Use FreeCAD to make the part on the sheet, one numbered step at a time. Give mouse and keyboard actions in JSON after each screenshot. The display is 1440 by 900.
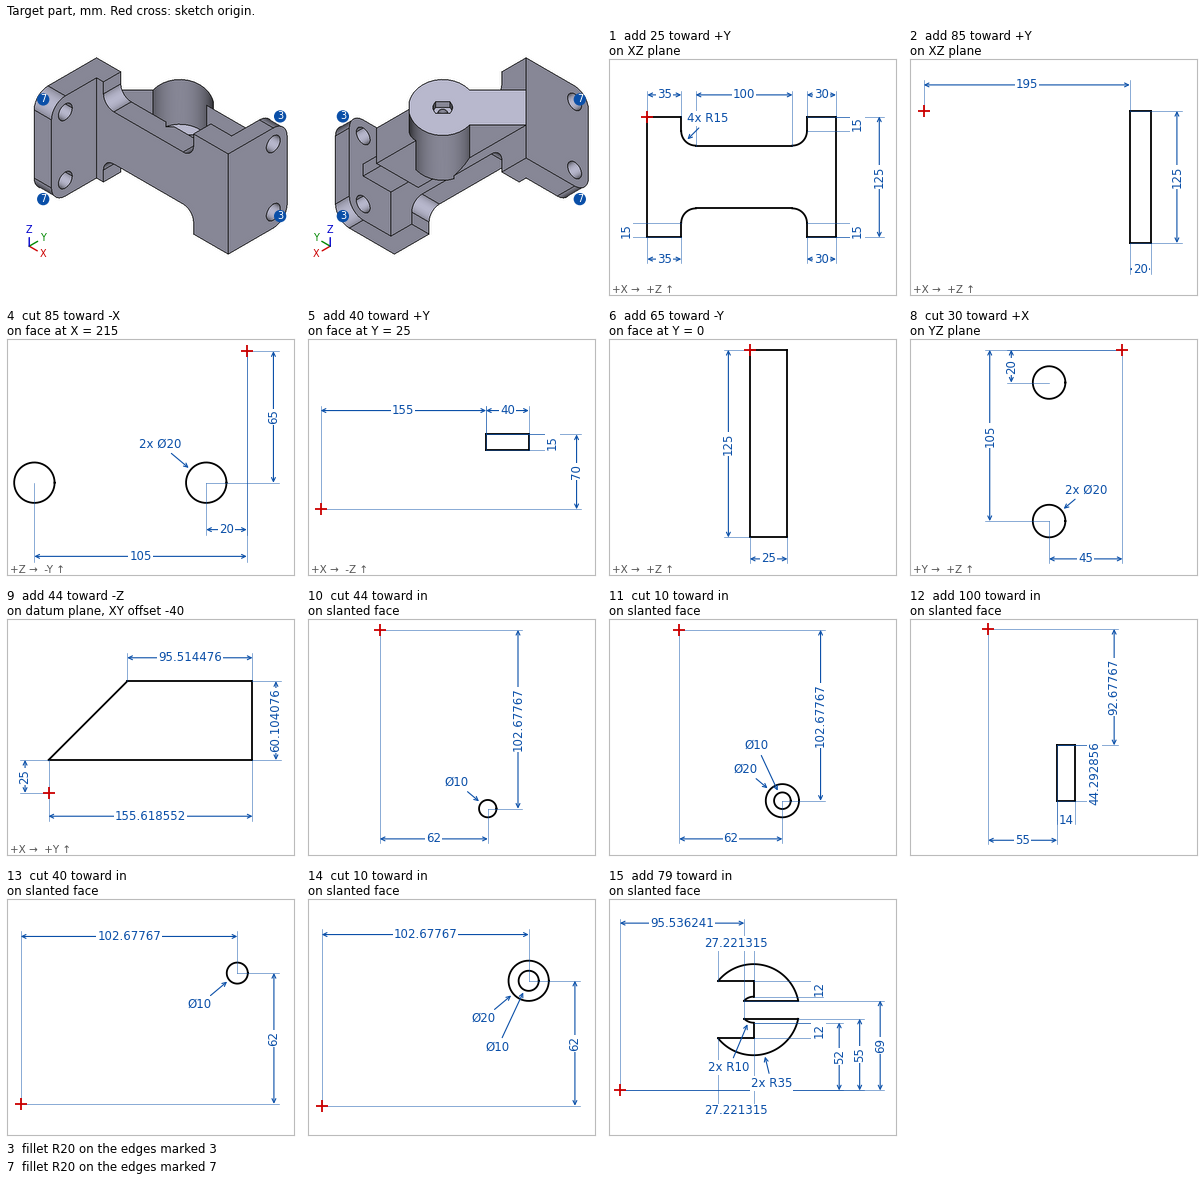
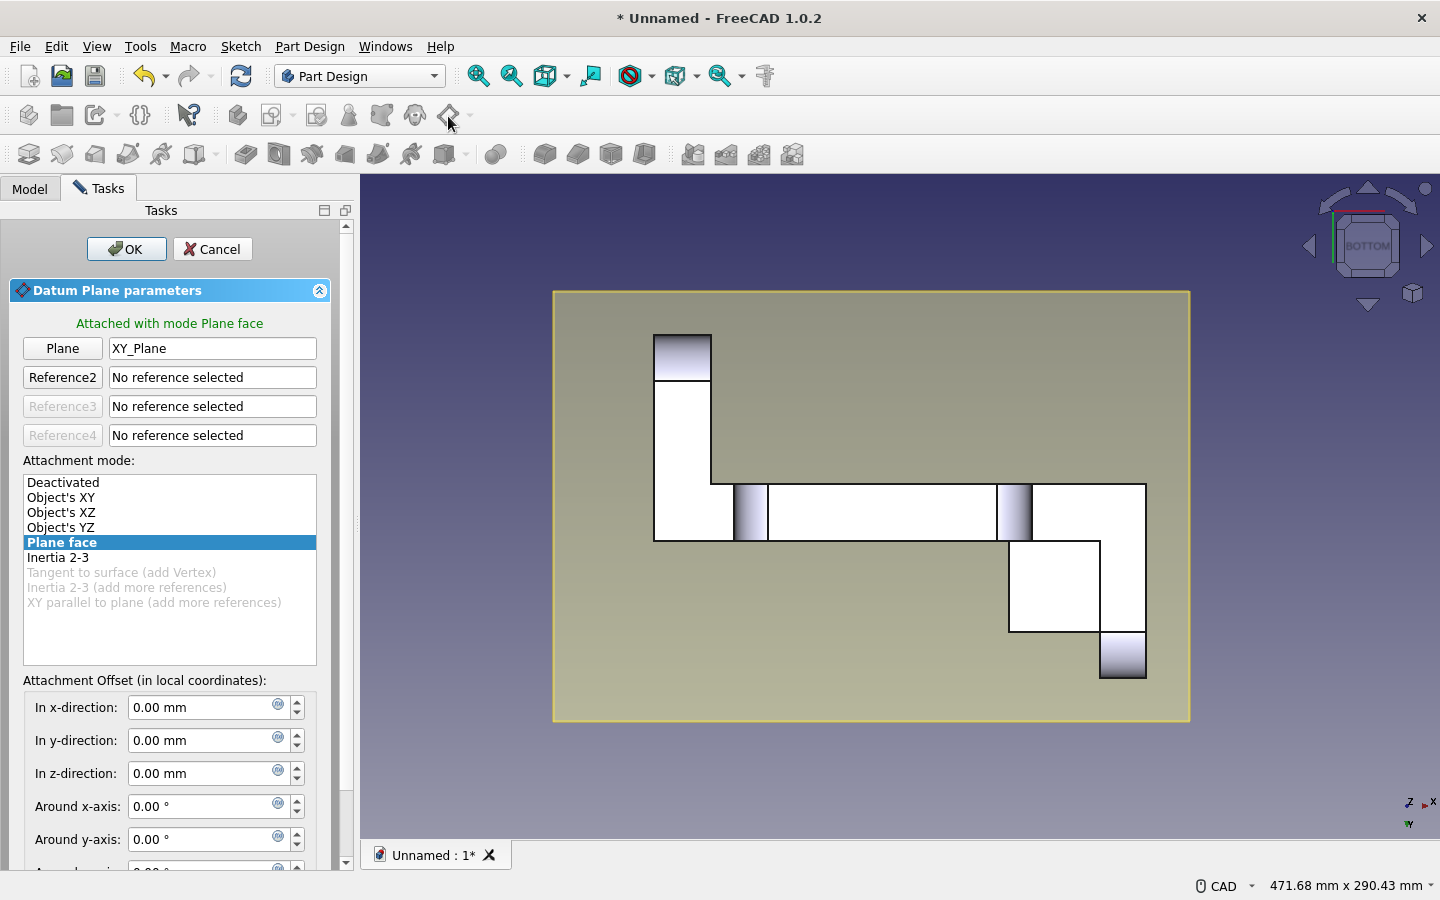
{"action": "triple_click", "coordinate": [210, 774]}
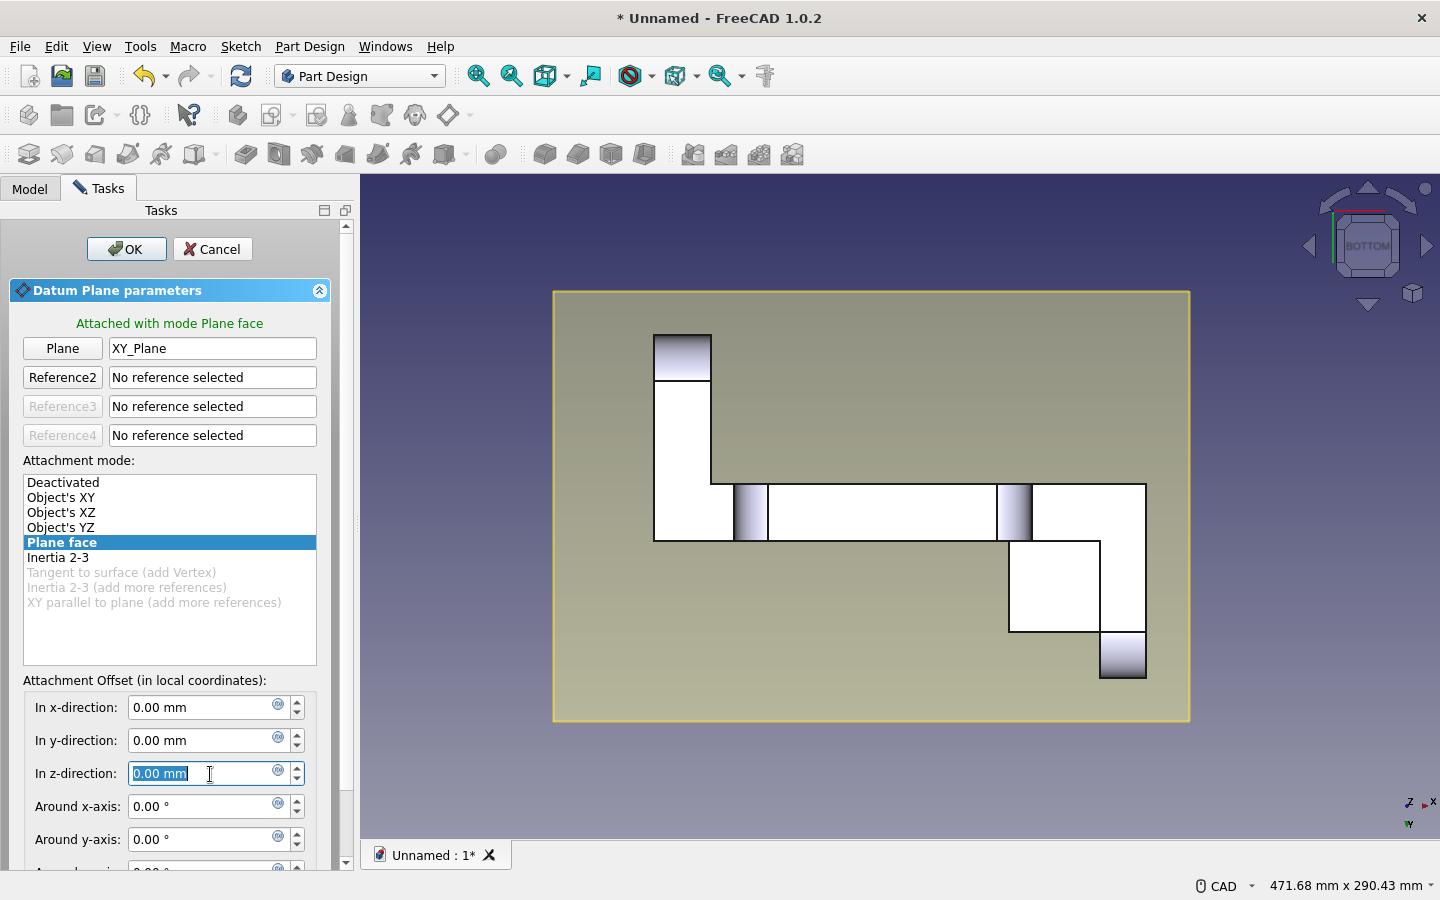
{"action": "type", "text": "-40"}
{"action": "key", "text": "Tab"}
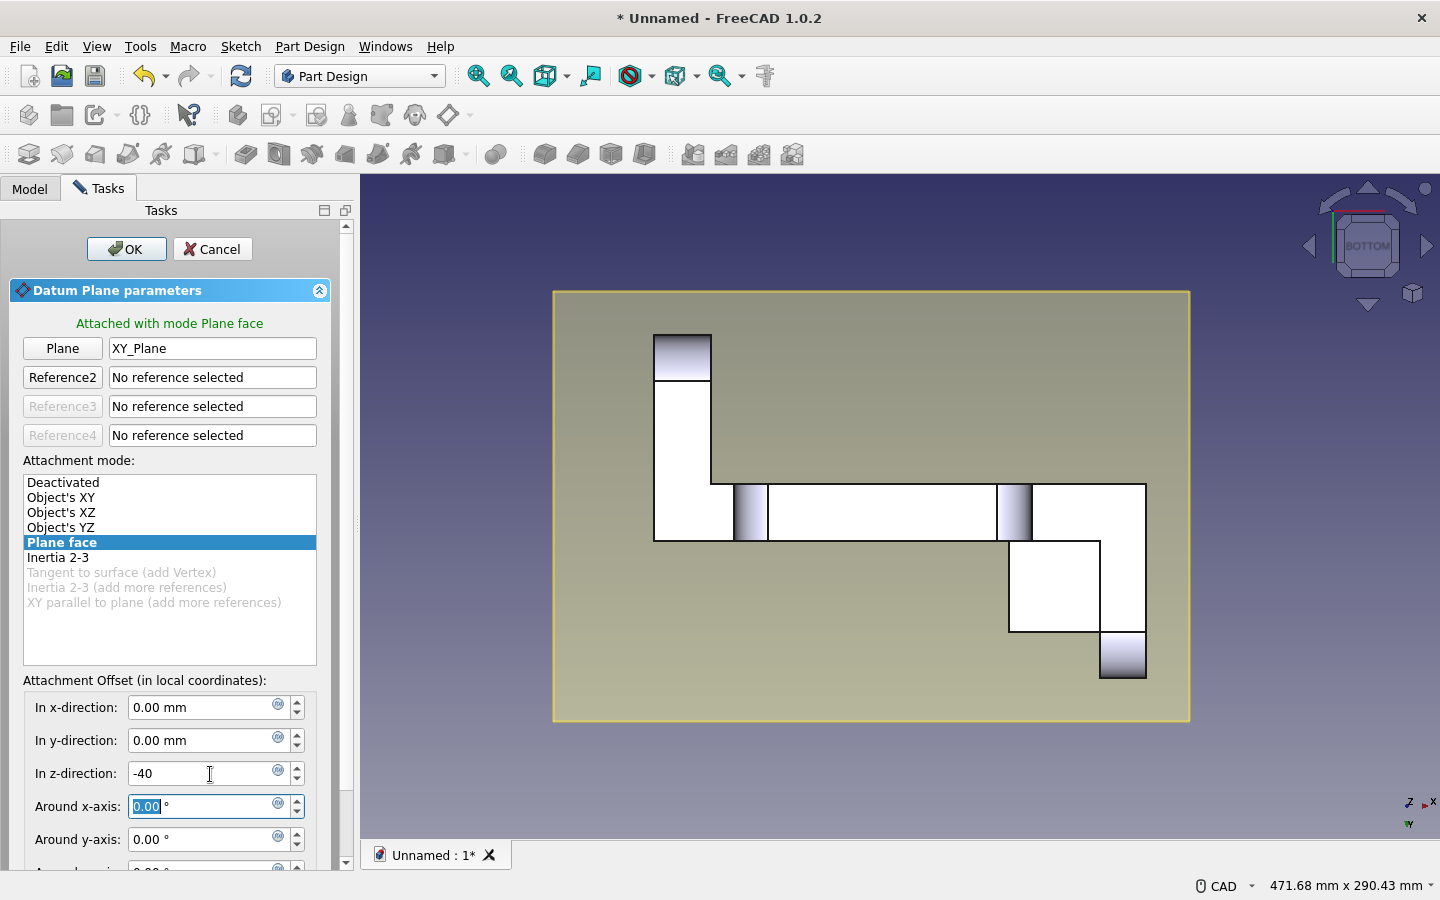
{"action": "left_click", "coordinate": [127, 249]}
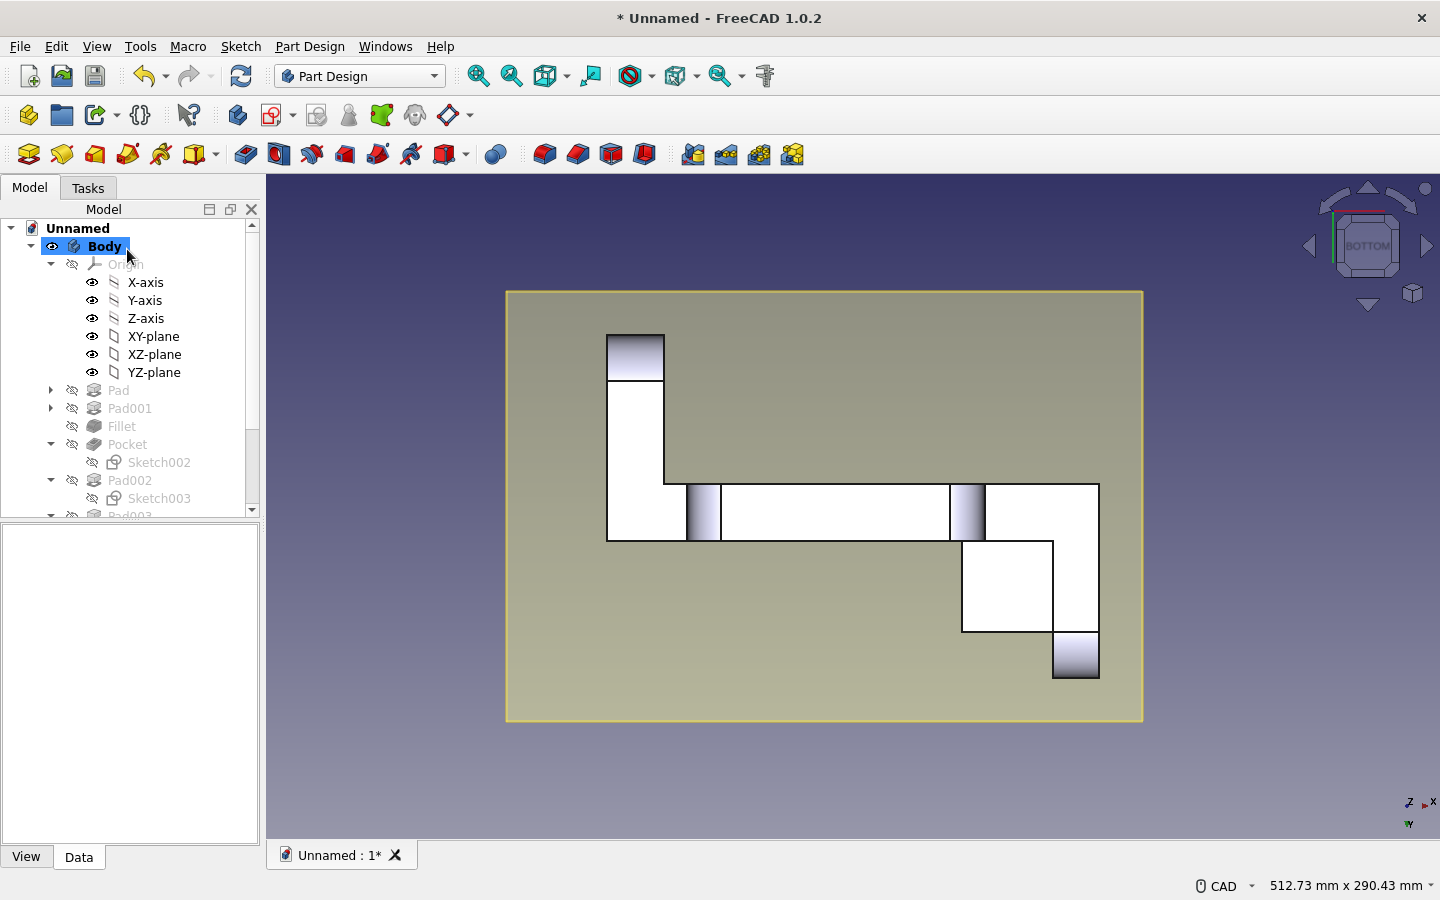
{"action": "scroll", "coordinate": [101, 368], "scroll_direction": "down", "scroll_amount": 3}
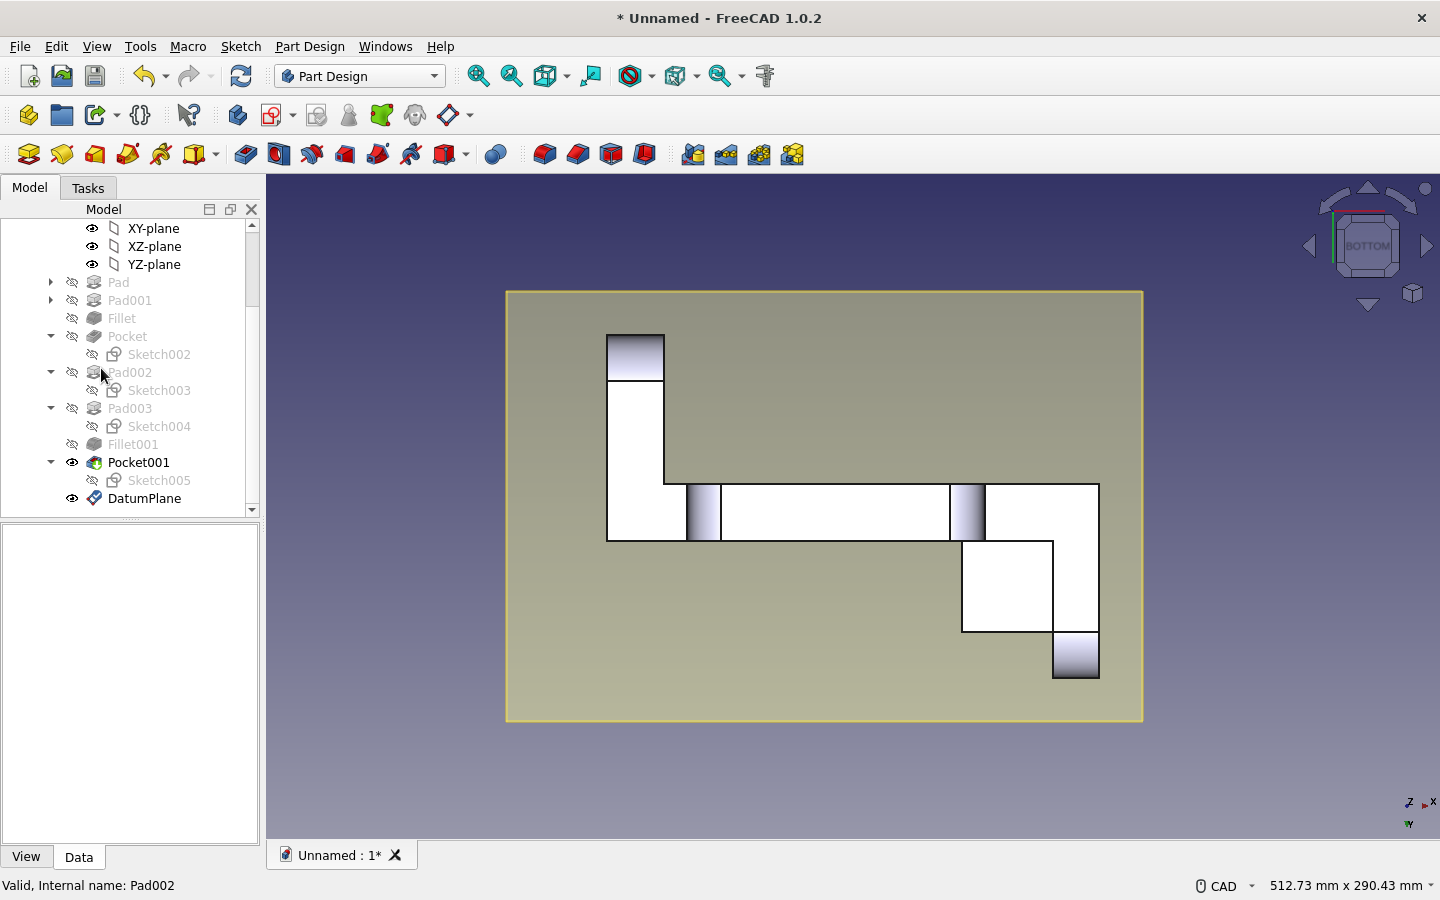
{"action": "left_click", "coordinate": [117, 498]}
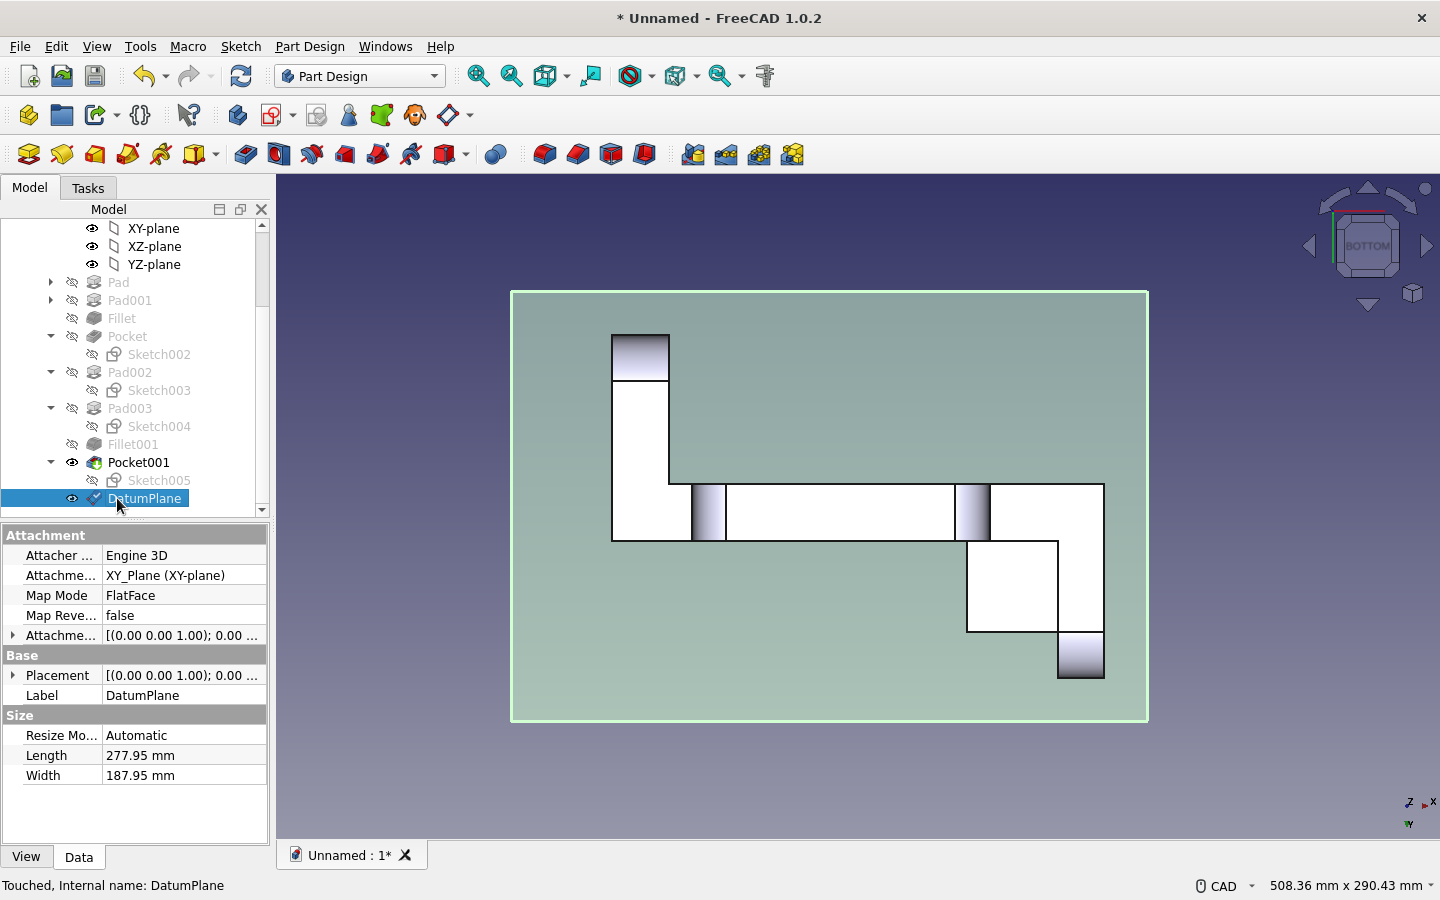
{"action": "left_click", "coordinate": [270, 116]}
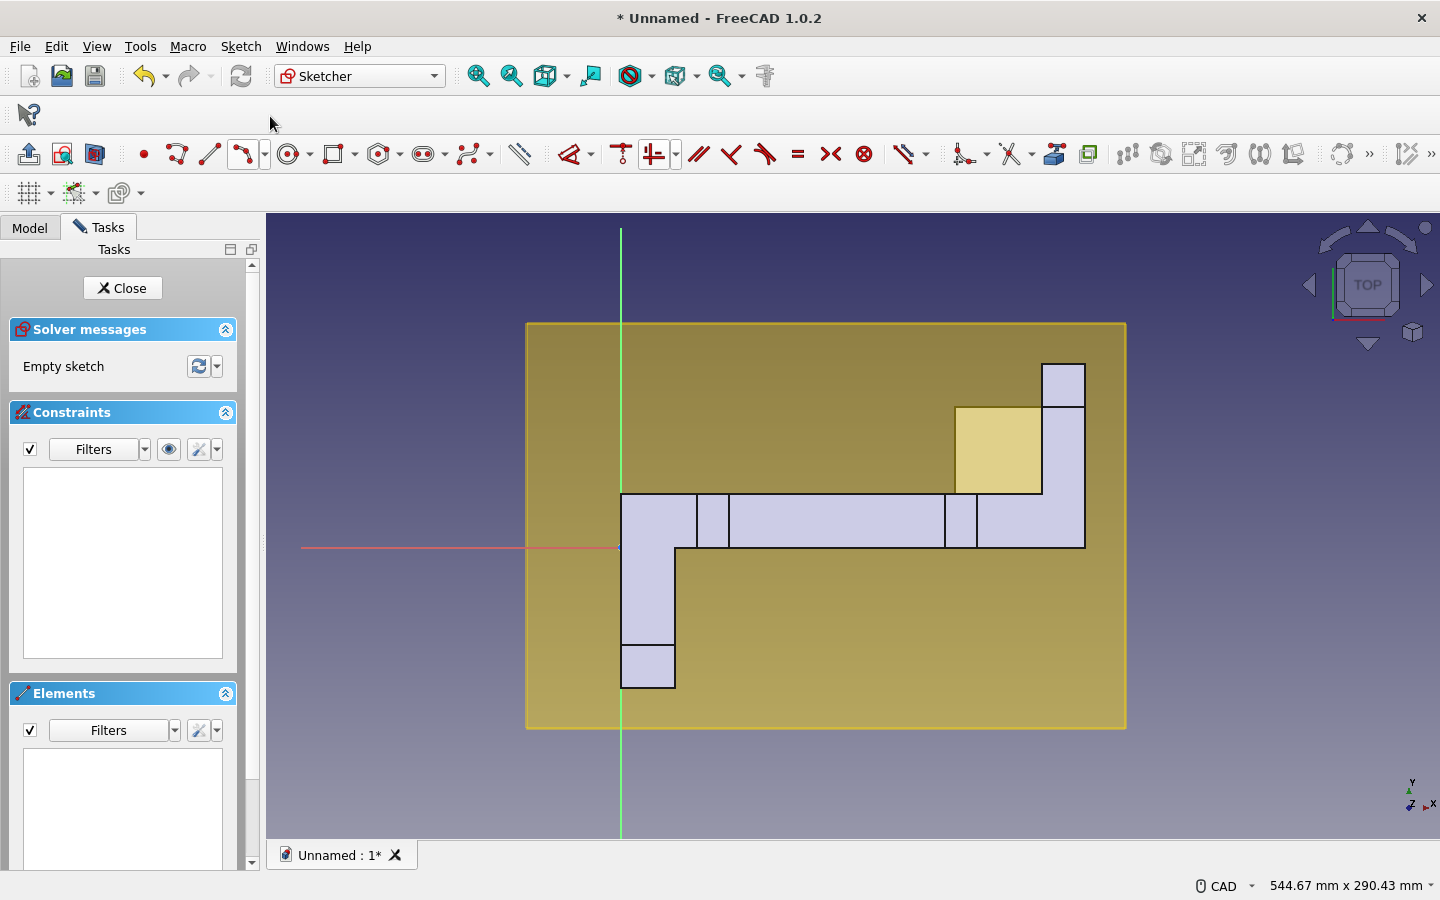
{"action": "key", "text": "q s"}